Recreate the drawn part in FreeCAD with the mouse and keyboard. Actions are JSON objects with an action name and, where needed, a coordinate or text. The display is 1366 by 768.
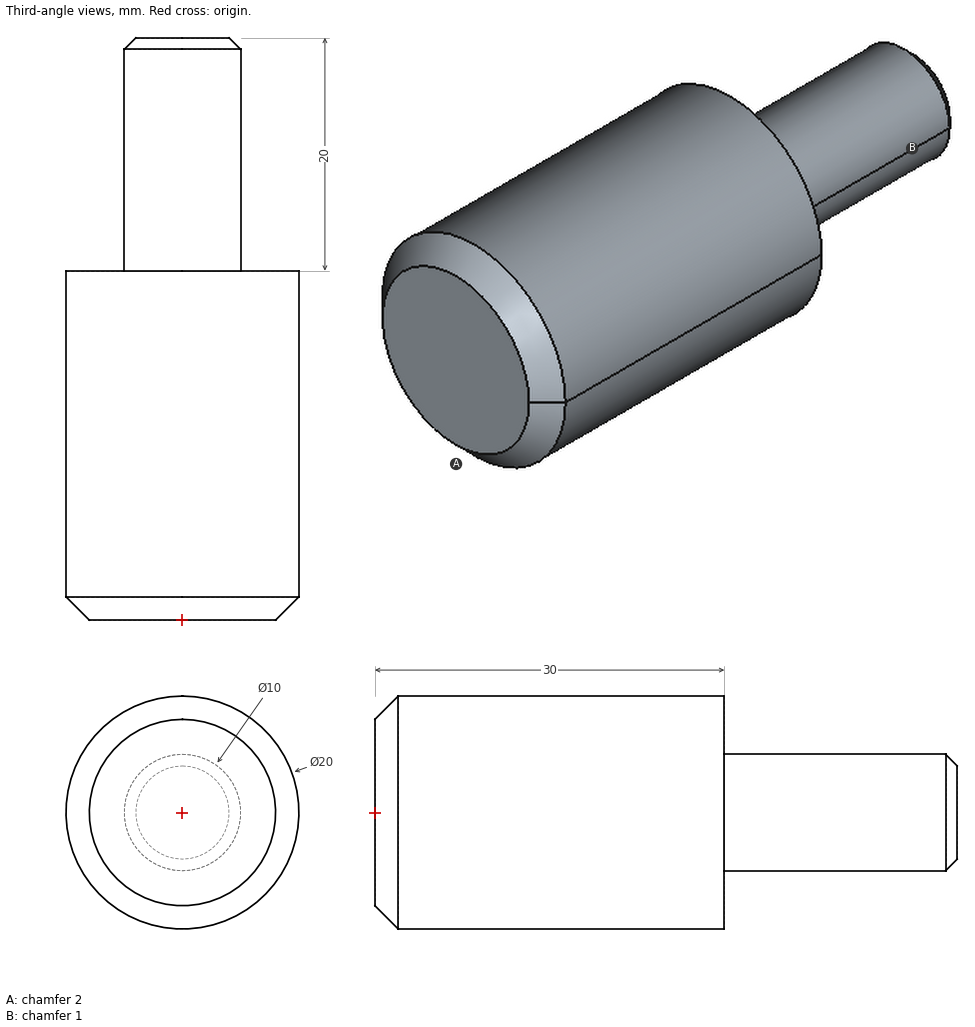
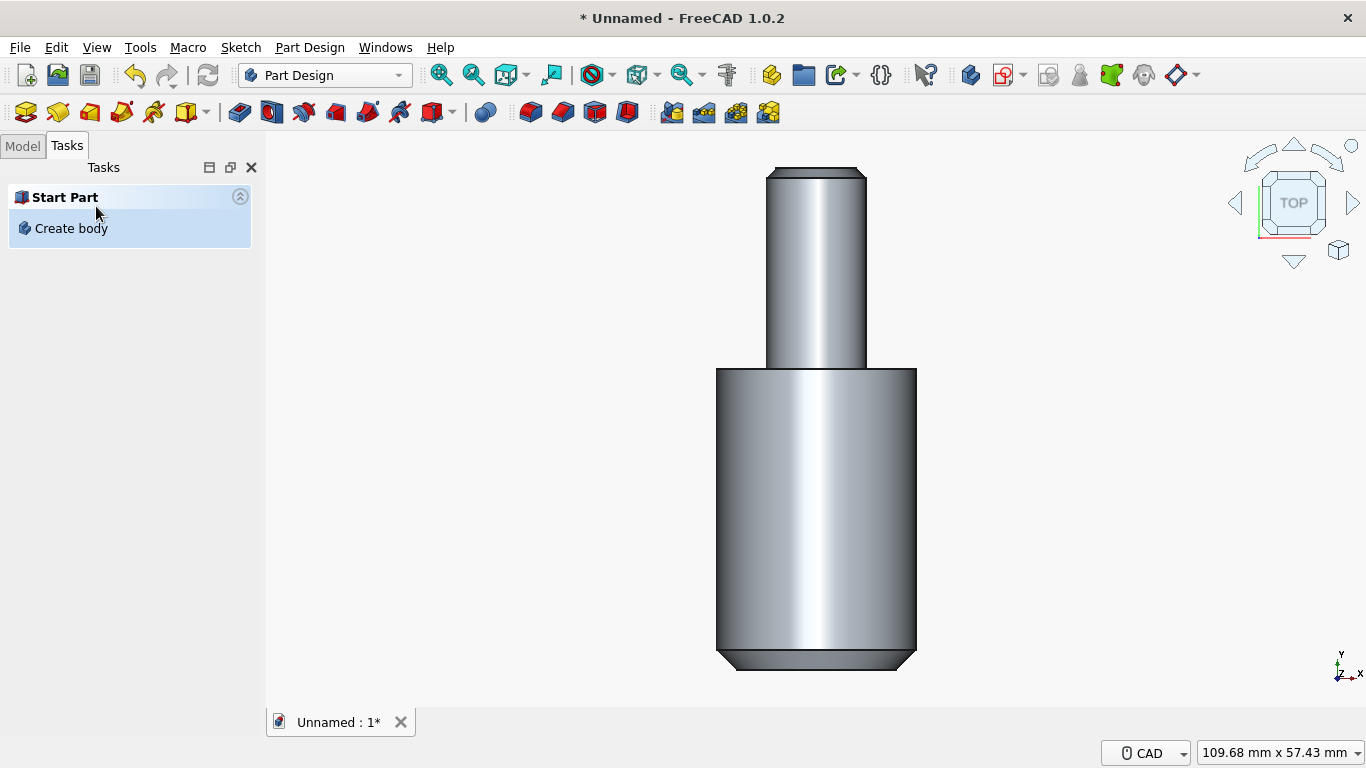
{"action": "key", "text": "0"}